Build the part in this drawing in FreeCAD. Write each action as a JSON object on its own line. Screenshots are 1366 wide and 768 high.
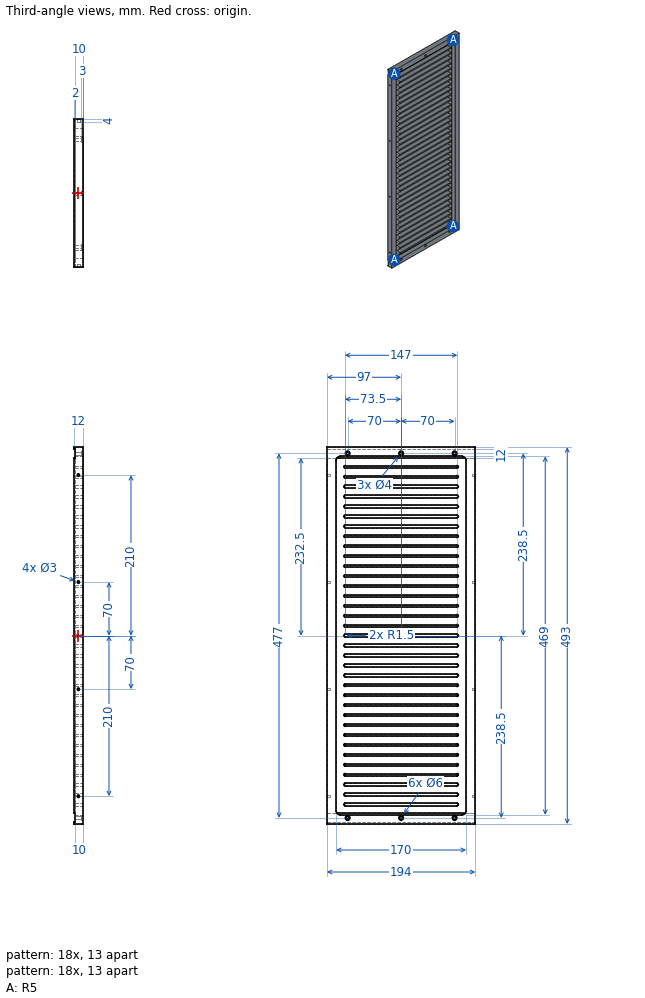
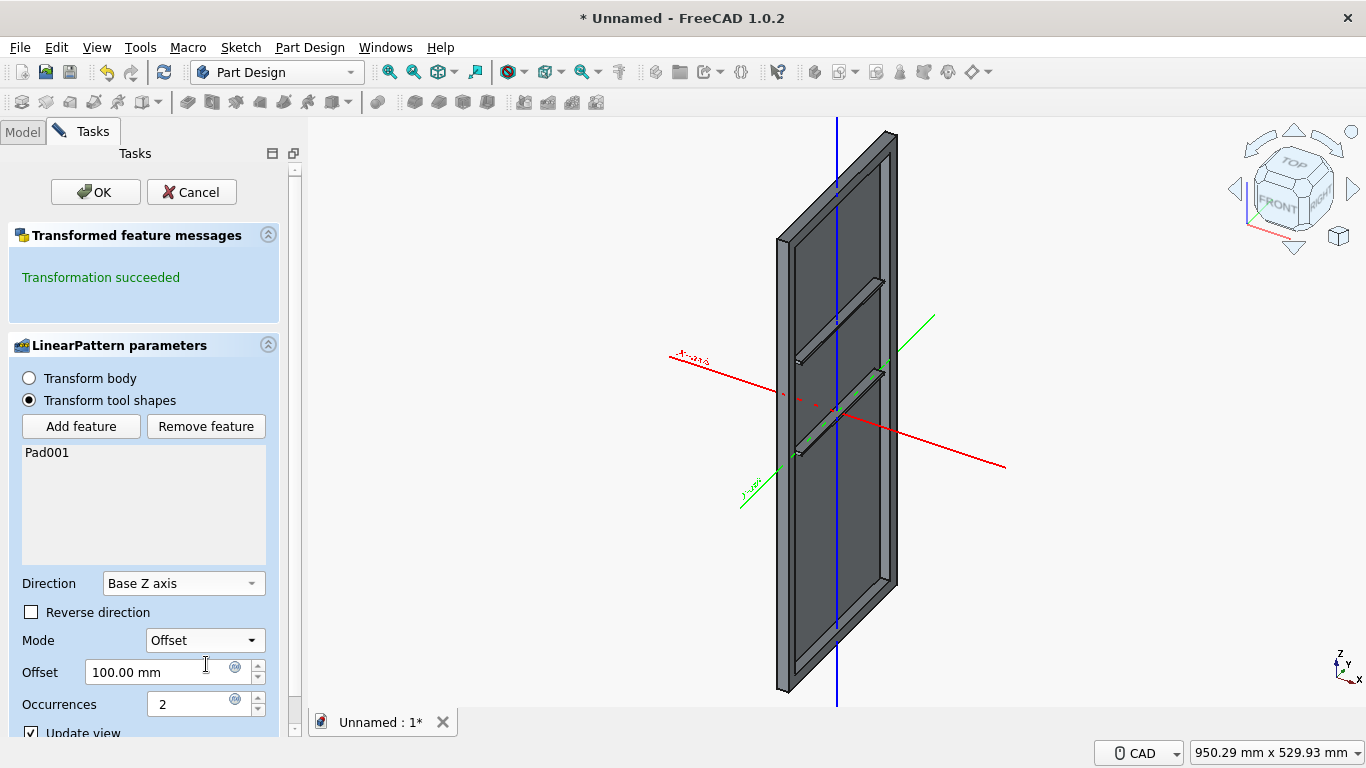
{"action": "triple_click", "coordinate": [168, 672]}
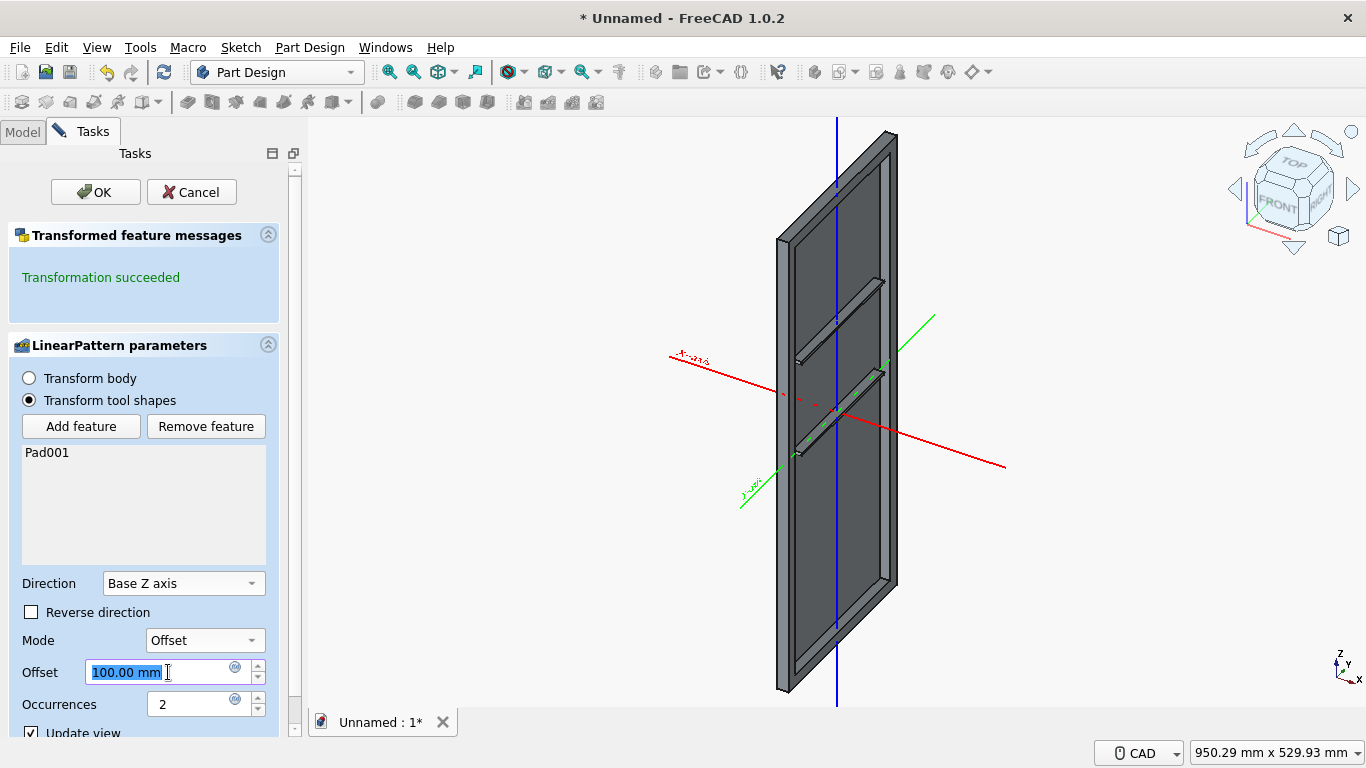
{"action": "type", "text": "13"}
{"action": "key", "text": "Tab"}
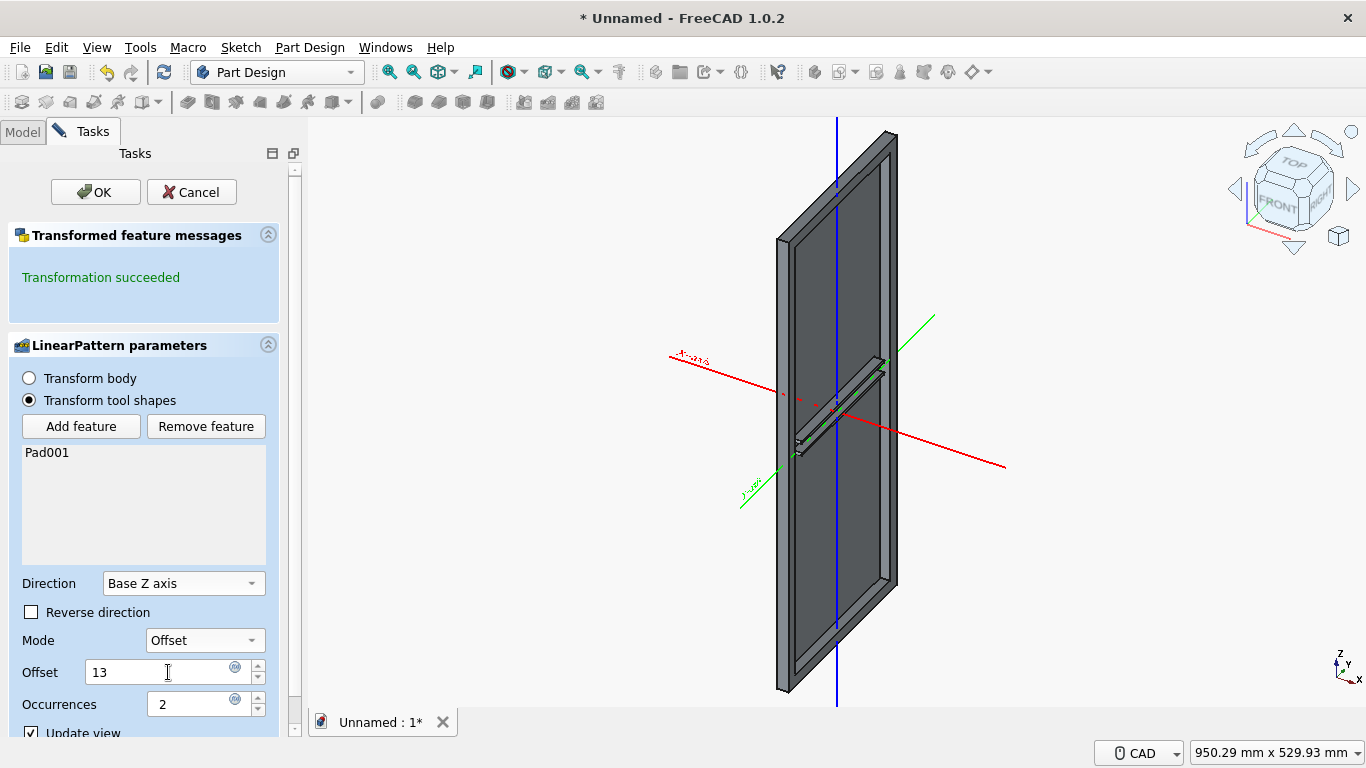
{"action": "triple_click", "coordinate": [198, 704]}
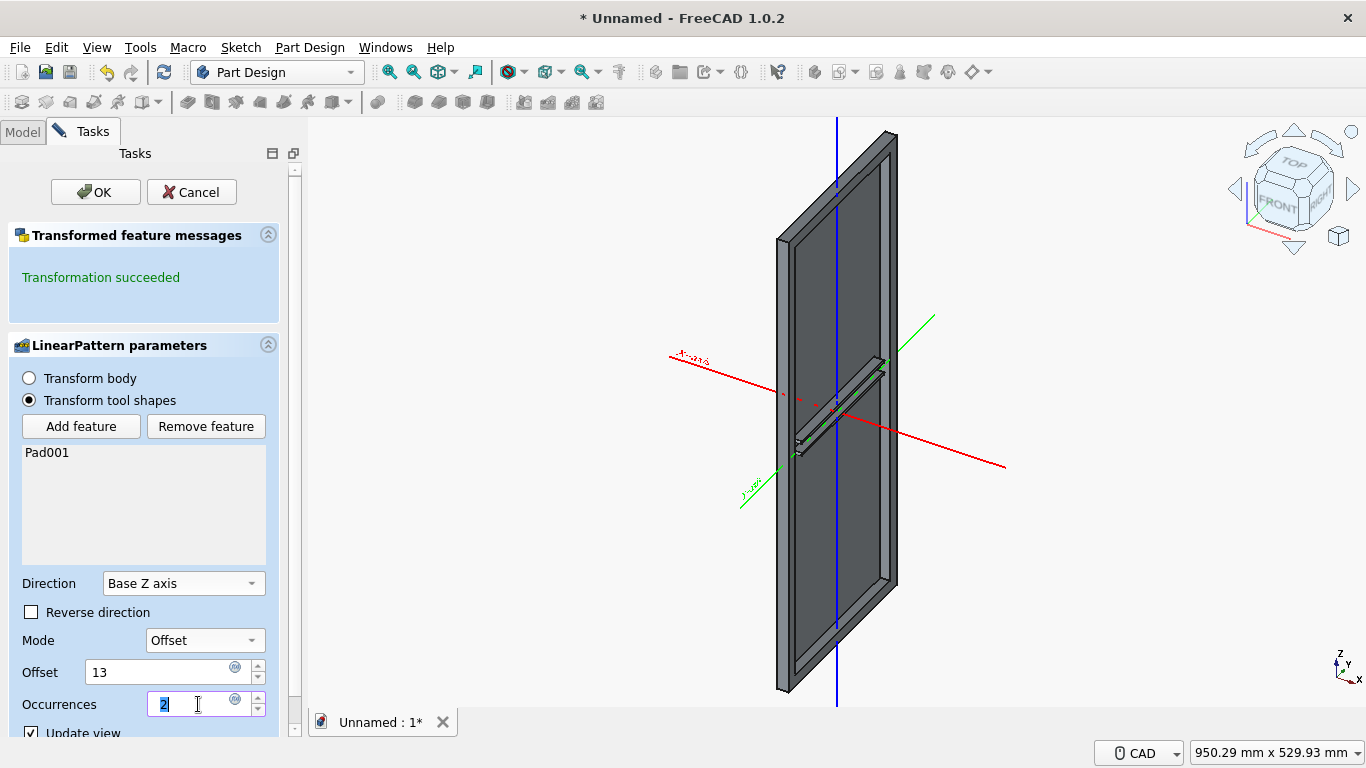
{"action": "type", "text": "18"}
{"action": "key", "text": "Tab"}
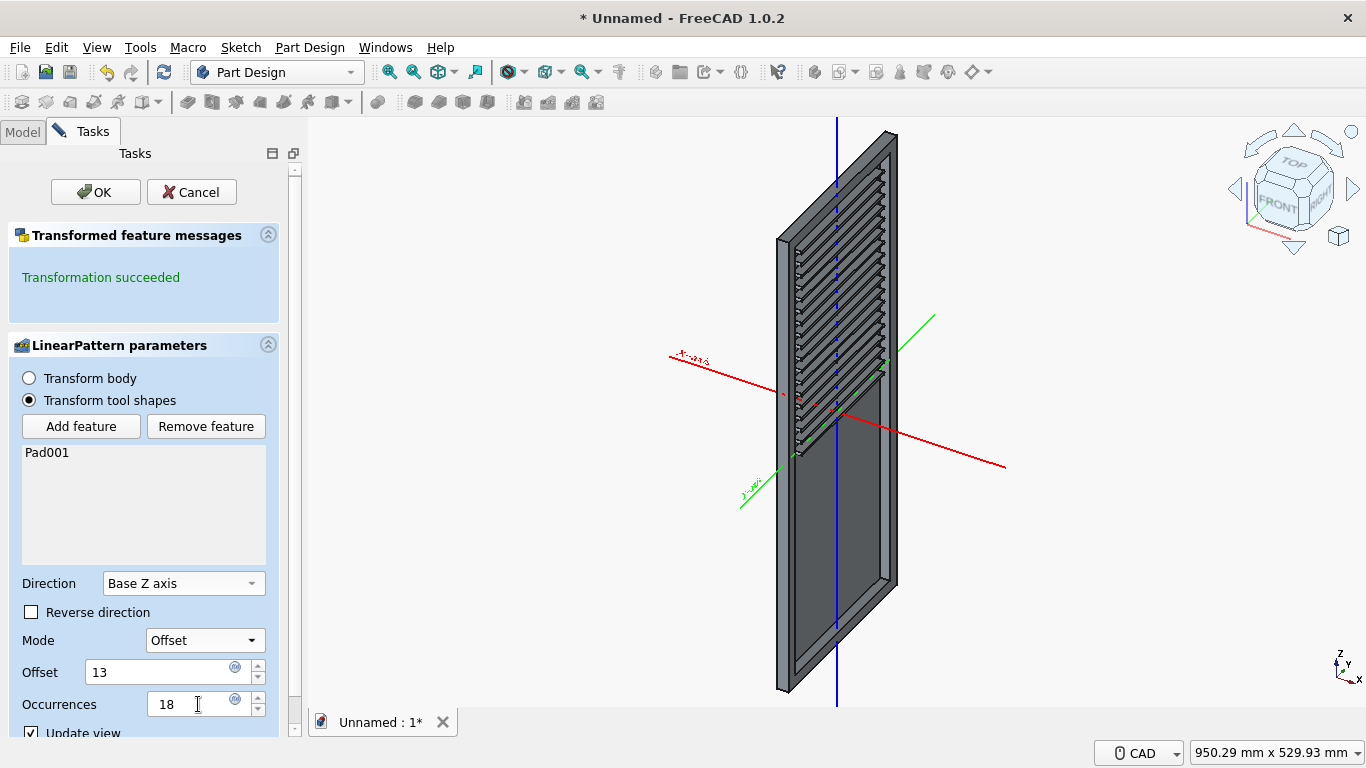
{"action": "left_click", "coordinate": [30, 612]}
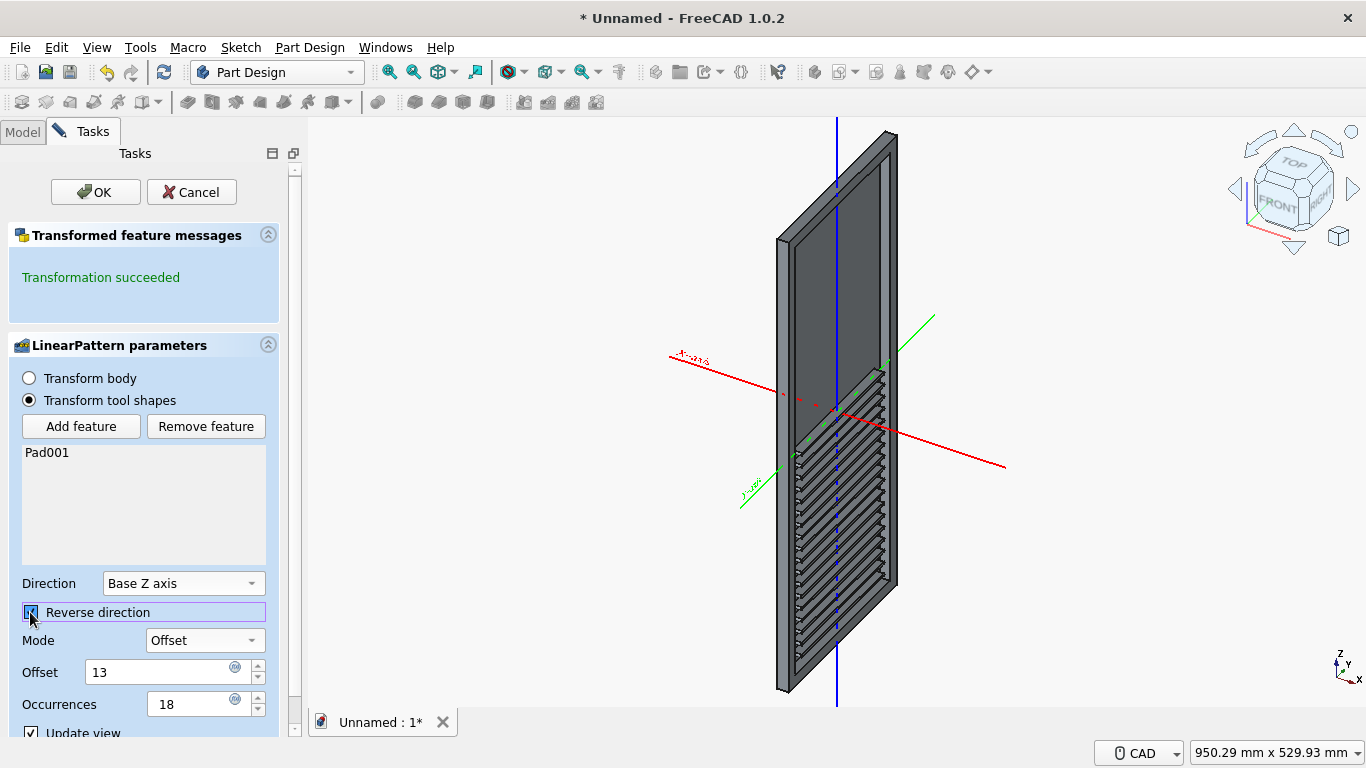
{"action": "left_click", "coordinate": [96, 192]}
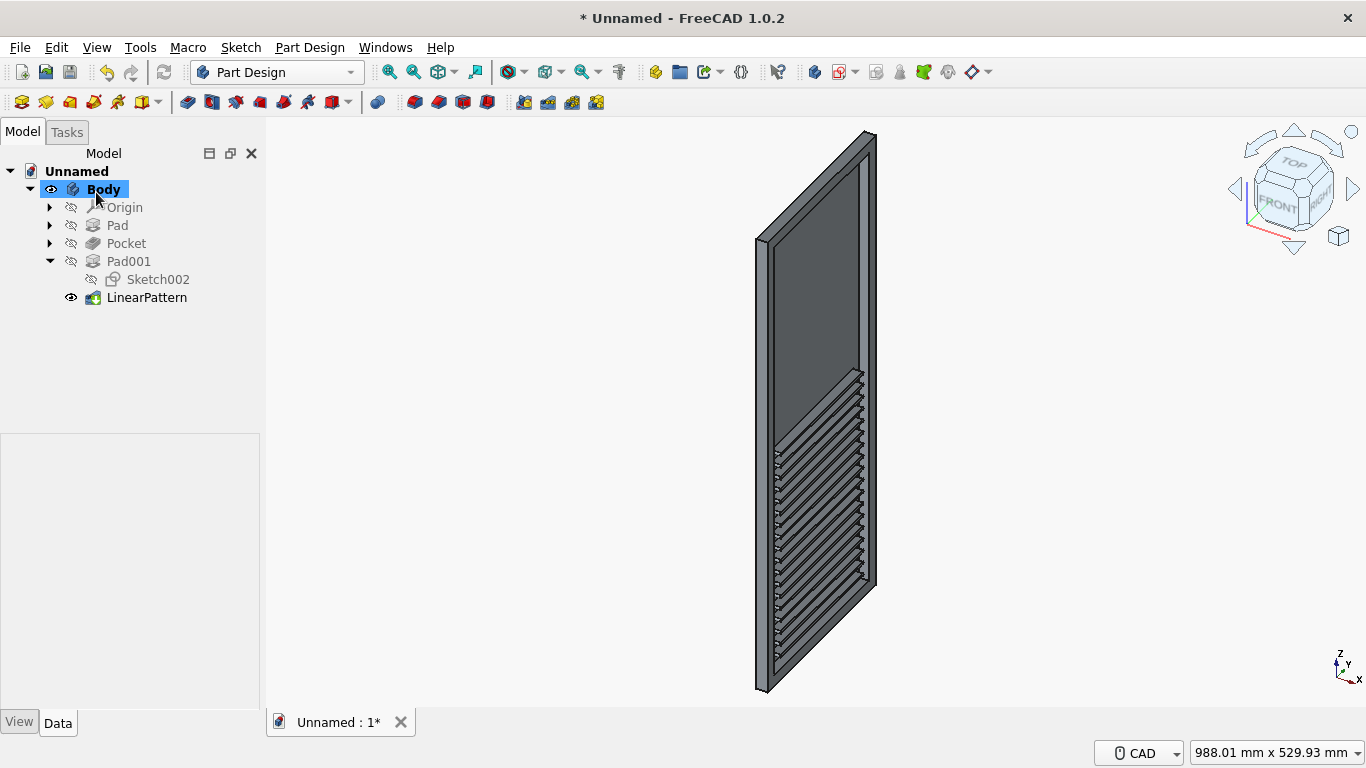
{"action": "left_click", "coordinate": [116, 261]}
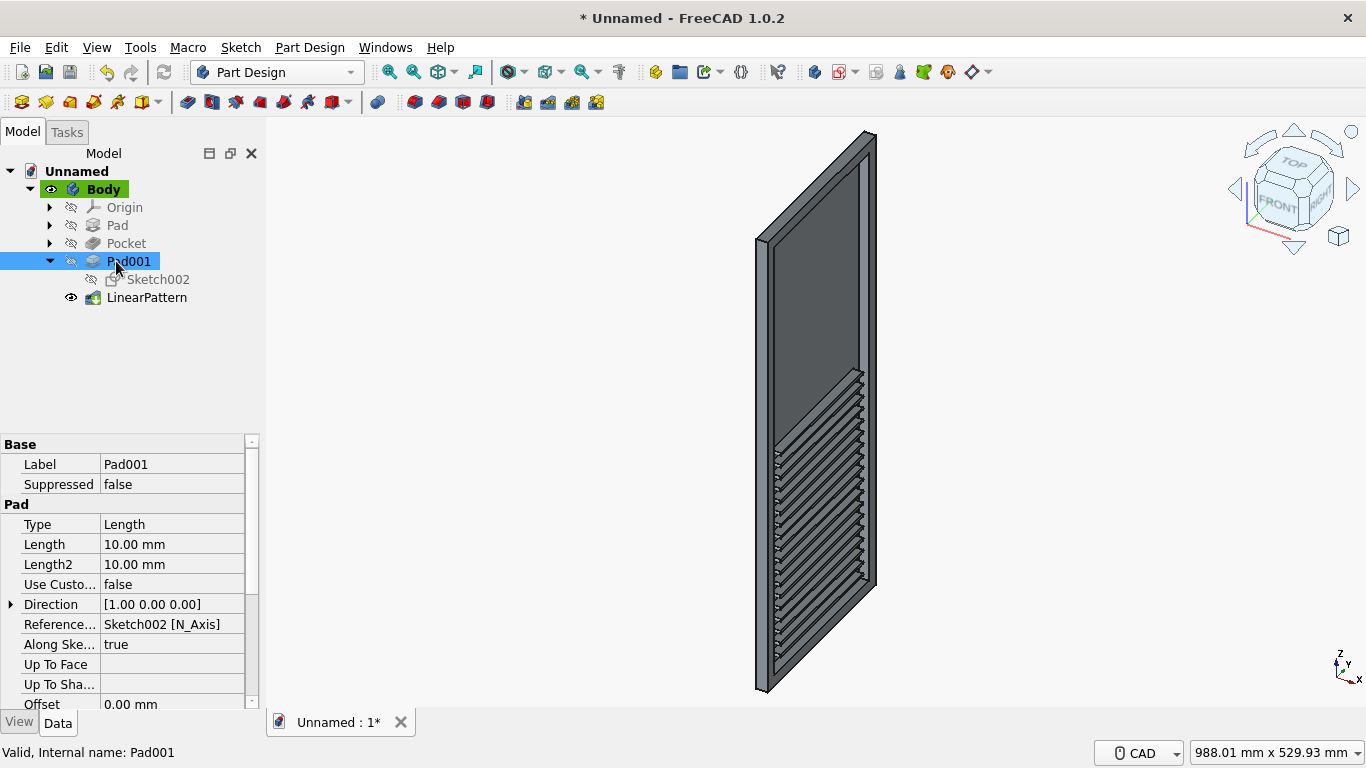
{"action": "left_click", "coordinate": [548, 102]}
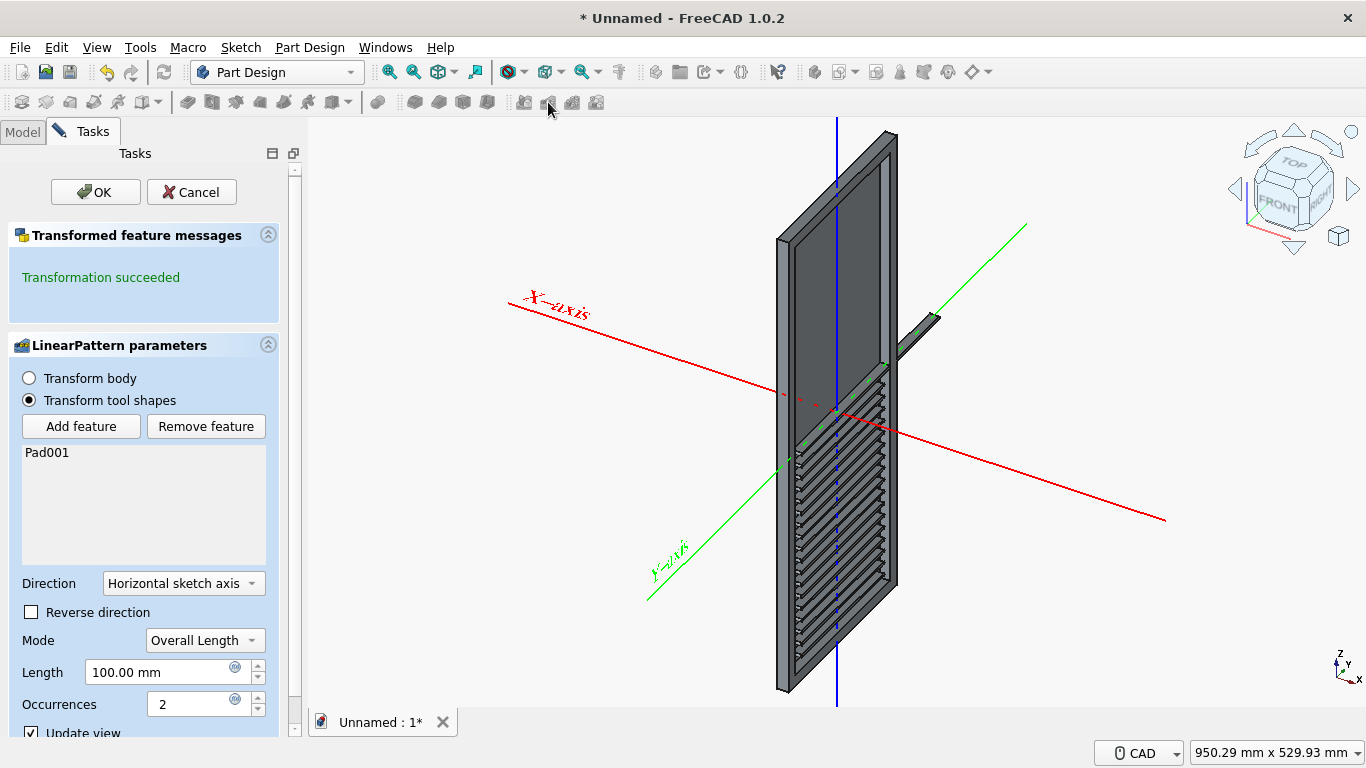
{"action": "left_click", "coordinate": [184, 584]}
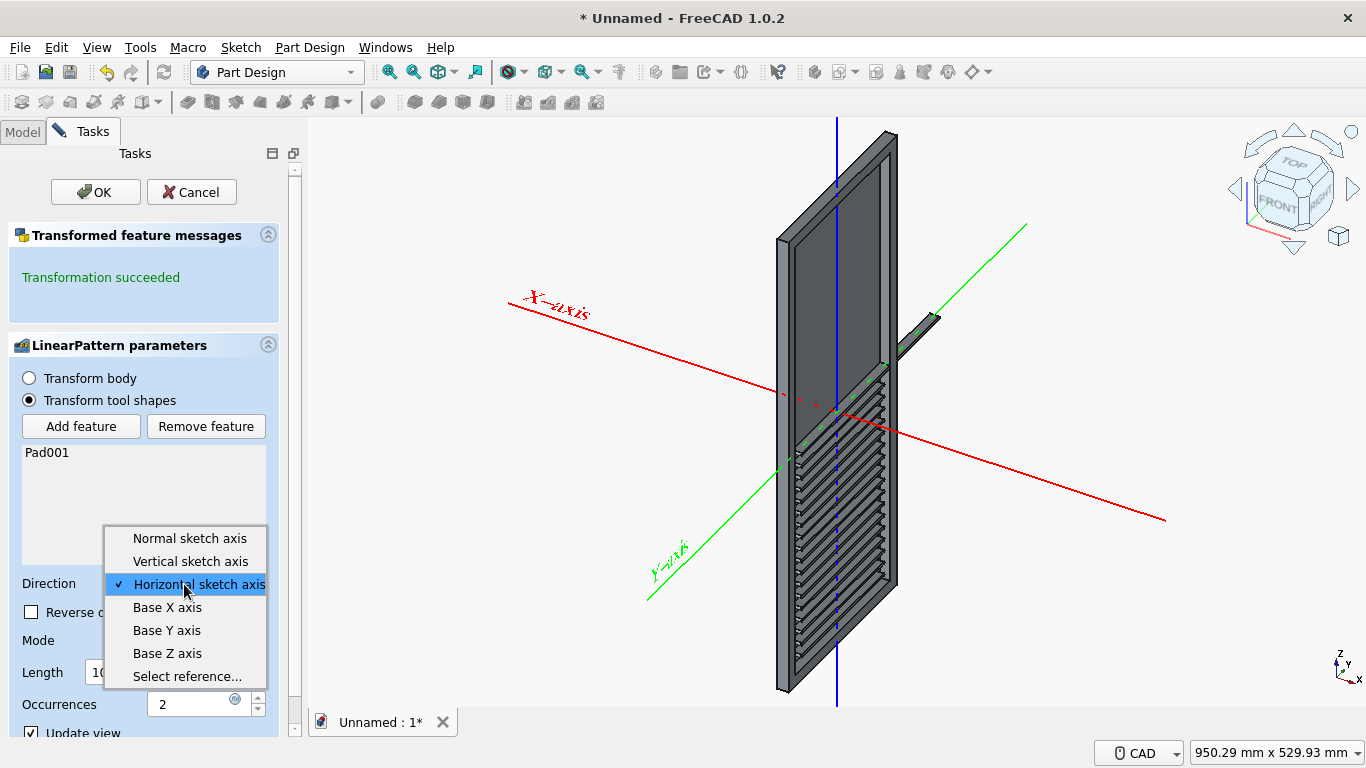
{"action": "left_click", "coordinate": [184, 654]}